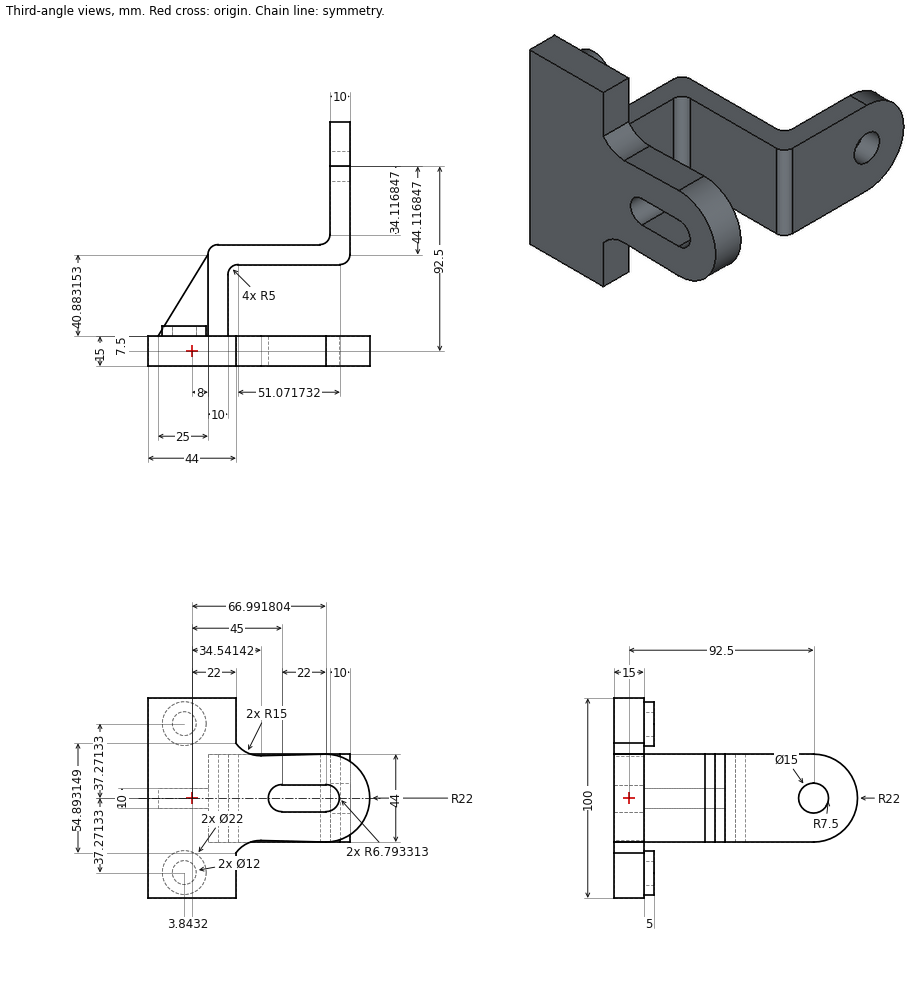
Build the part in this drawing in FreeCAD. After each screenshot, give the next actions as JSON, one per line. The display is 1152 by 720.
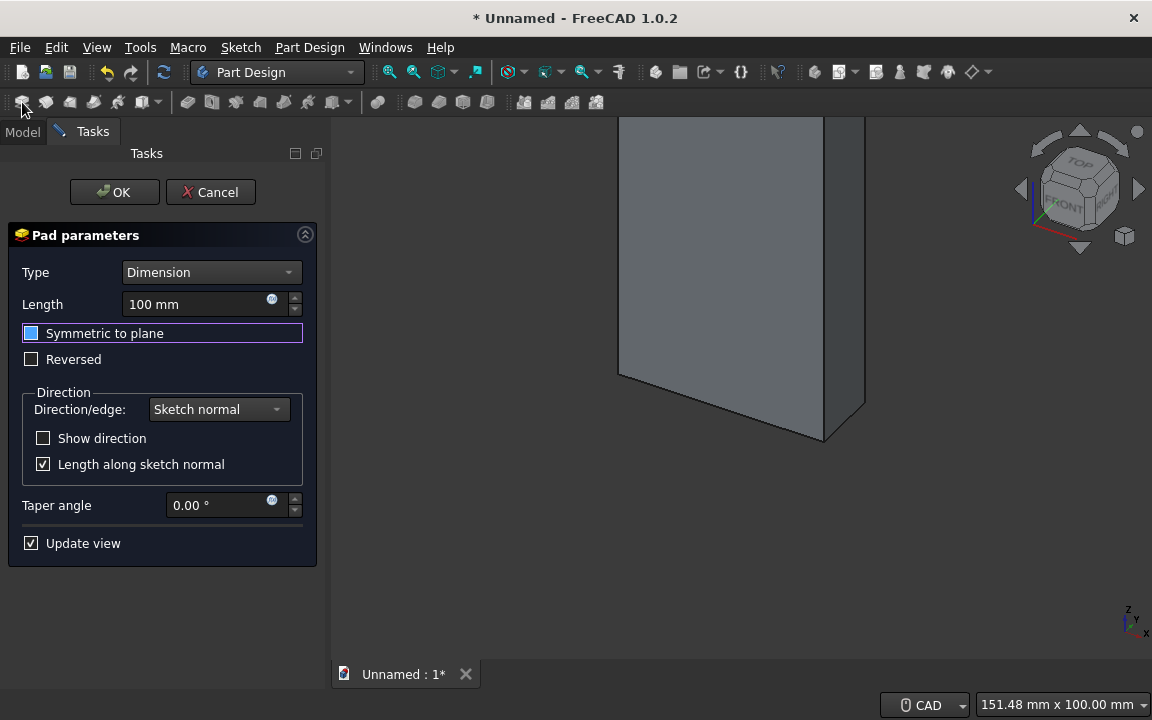
{"action": "left_click", "coordinate": [30, 333]}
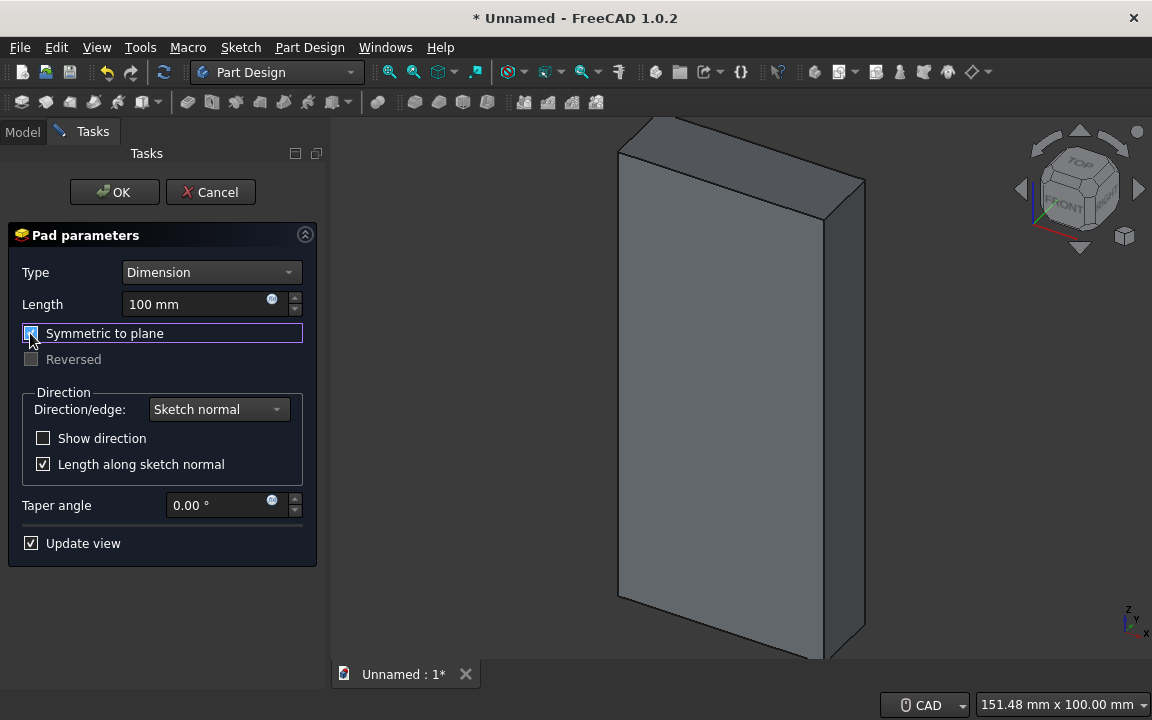
{"action": "left_click", "coordinate": [115, 192]}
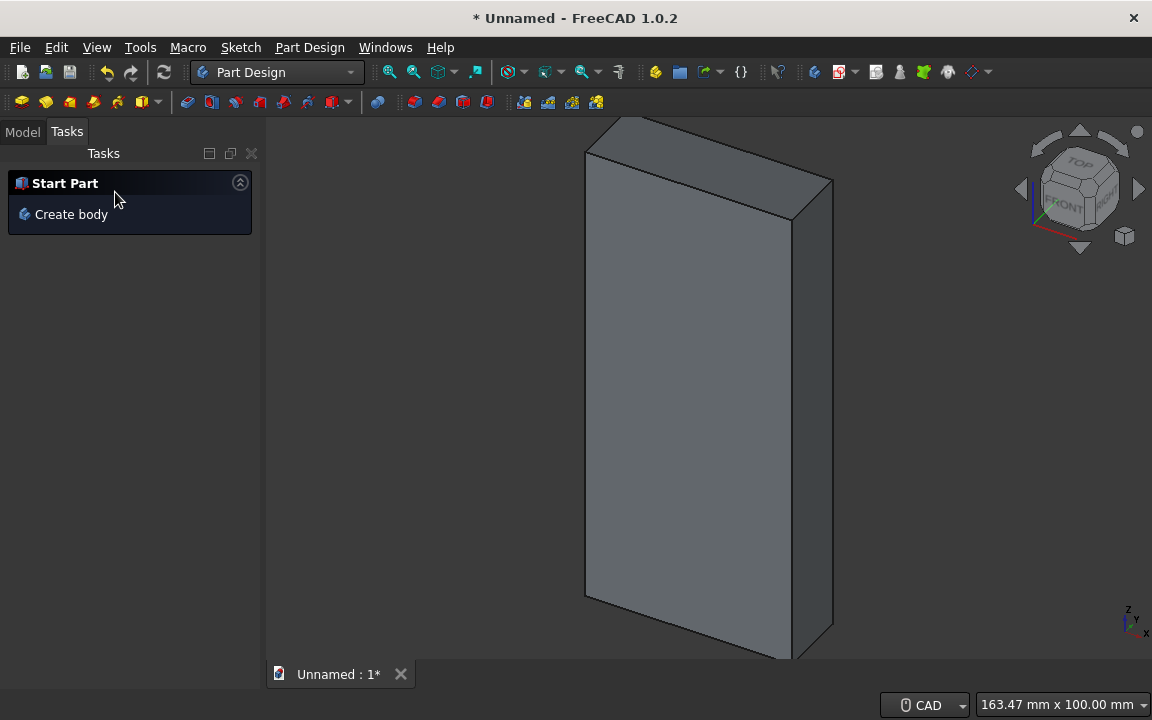
{"action": "left_click", "coordinate": [390, 72]}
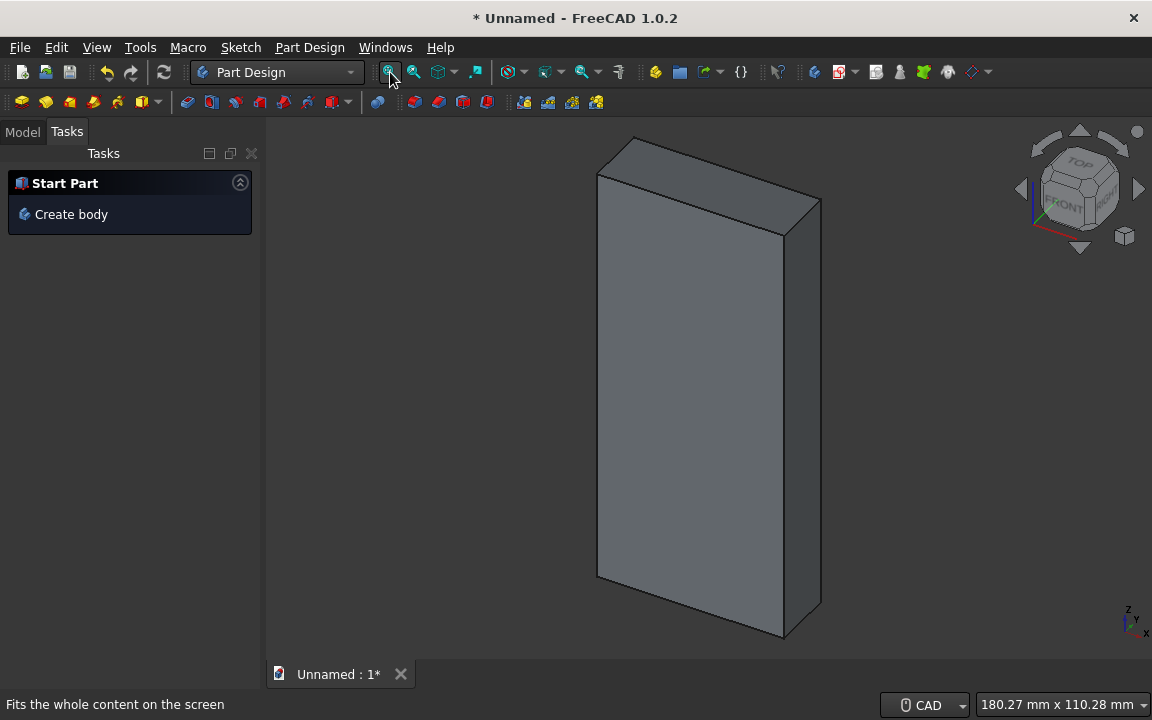
{"action": "left_click", "coordinate": [840, 72]}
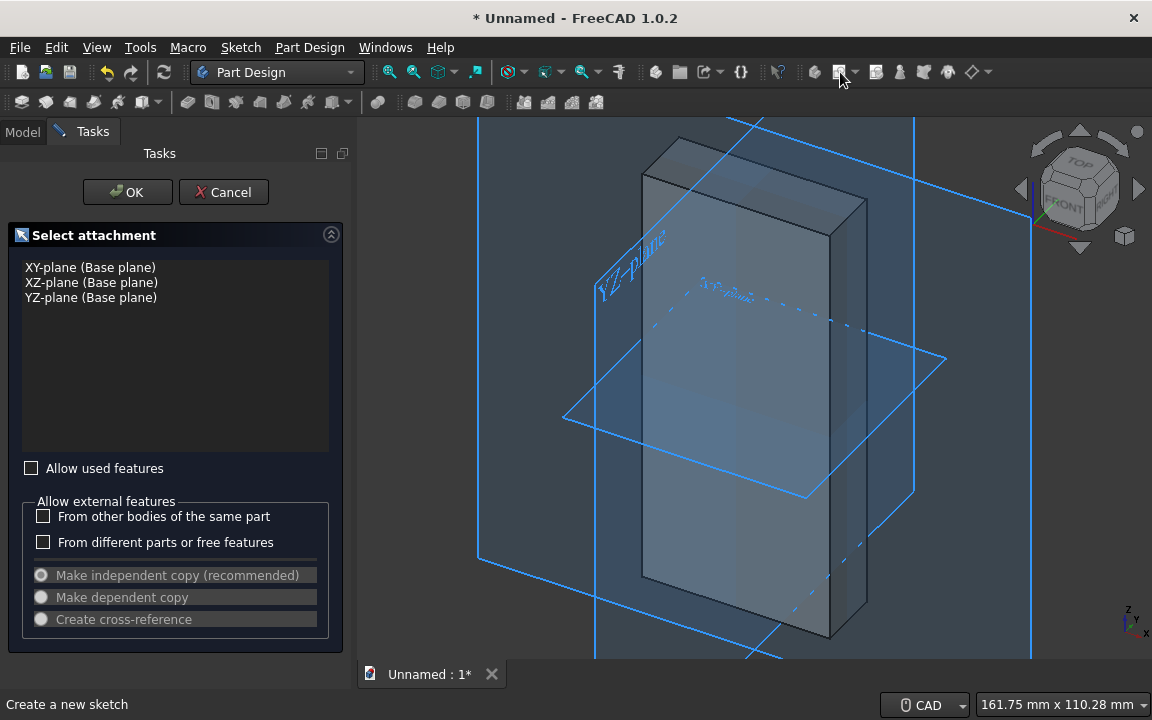
{"action": "left_click", "coordinate": [82, 268]}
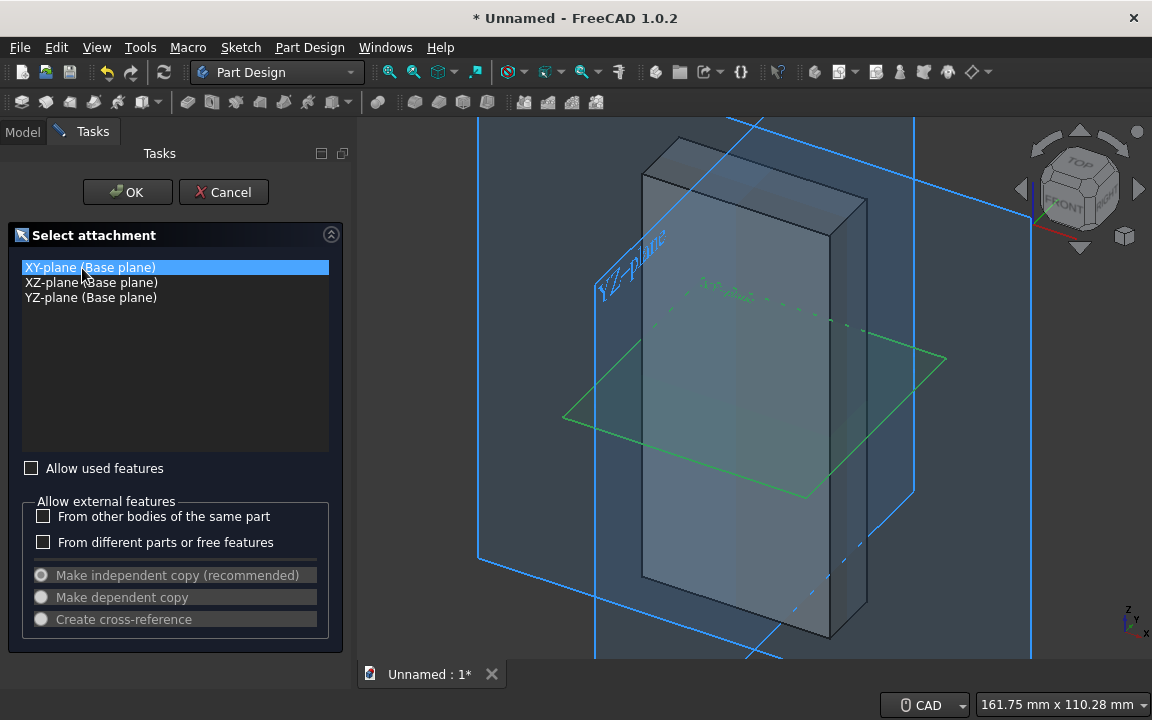
{"action": "left_click", "coordinate": [128, 192]}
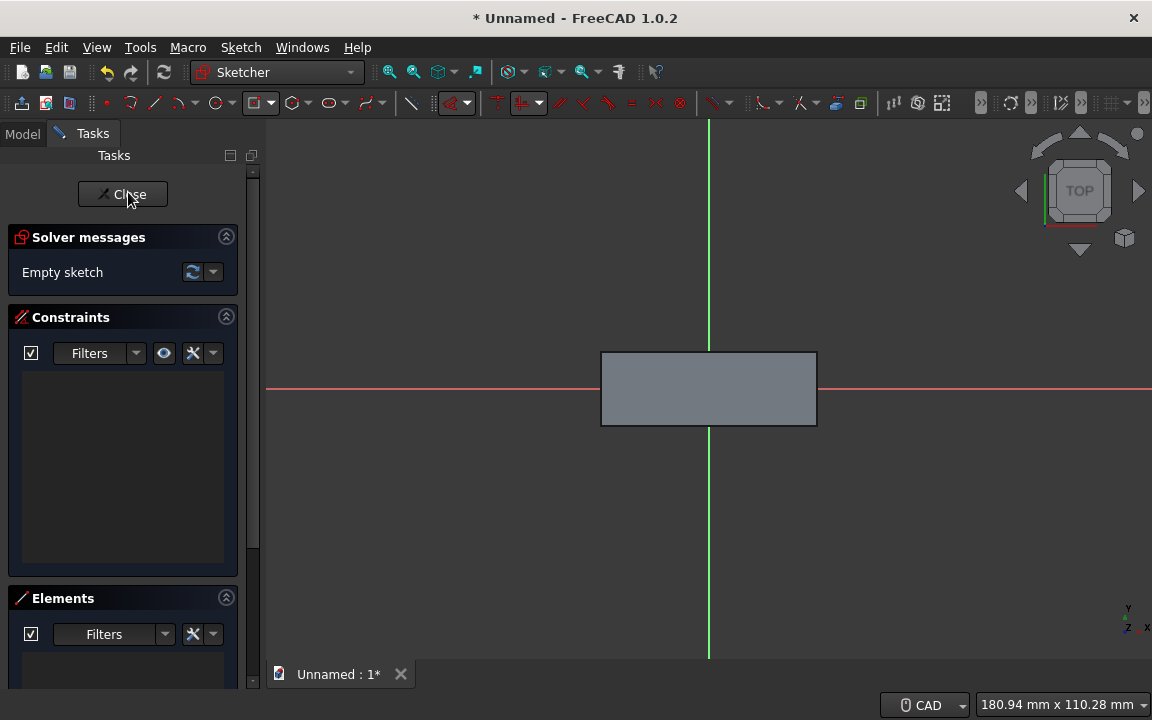
{"action": "left_click", "coordinate": [70, 104]}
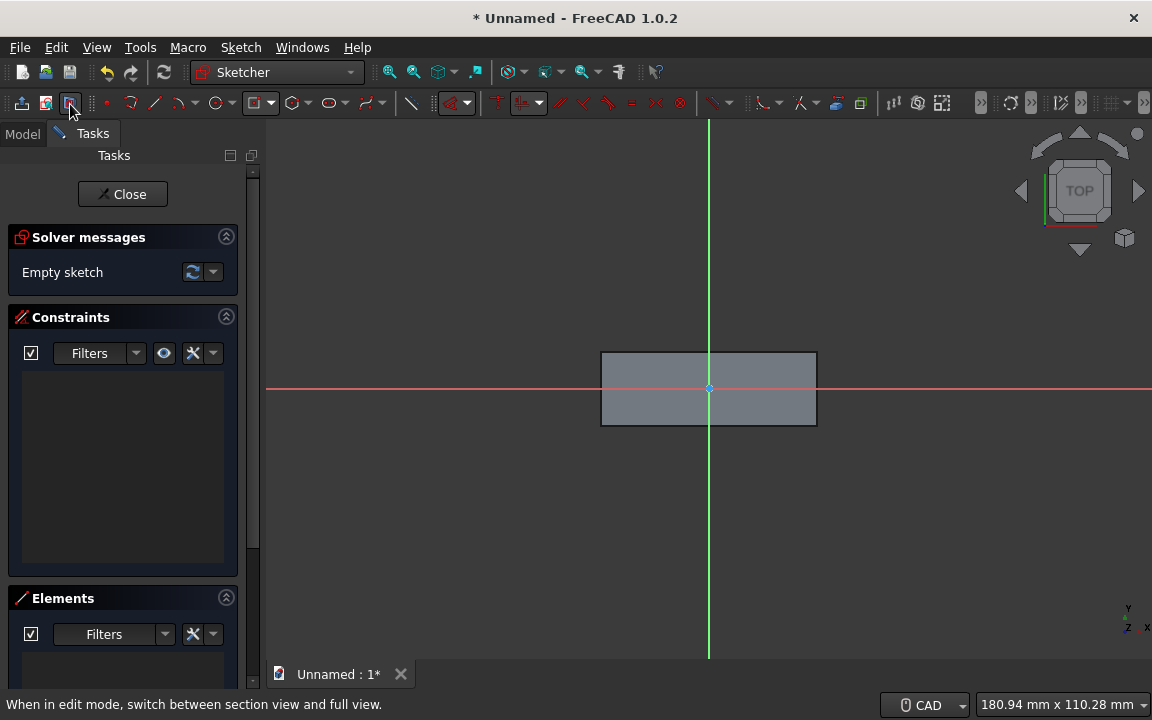
{"action": "scroll", "coordinate": [322, 631], "scroll_direction": "down", "scroll_amount": 3}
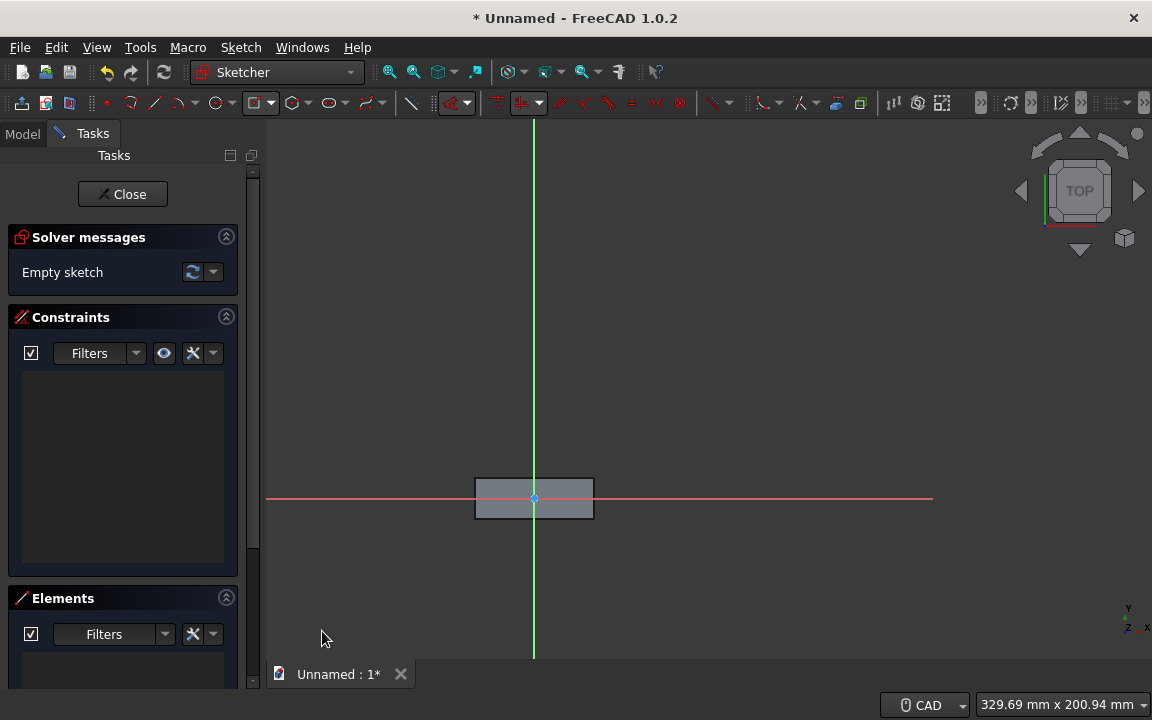
{"action": "scroll", "coordinate": [641, 344], "scroll_direction": "up", "scroll_amount": 2}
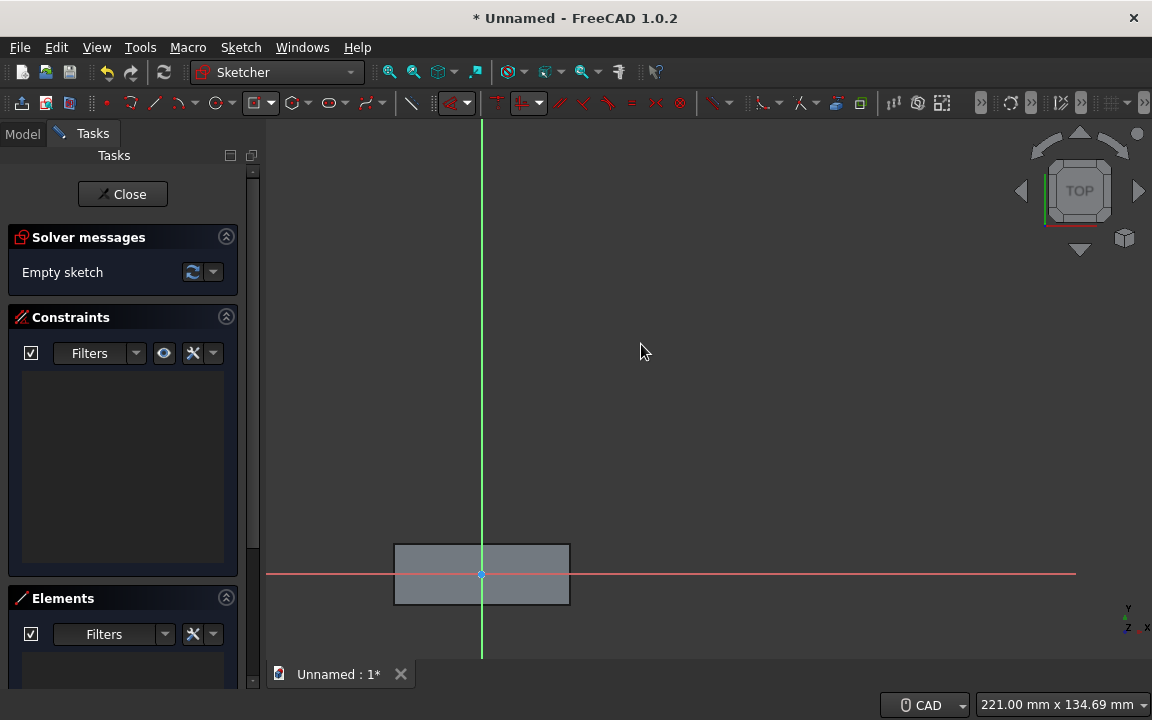
{"action": "left_click", "coordinate": [156, 104]}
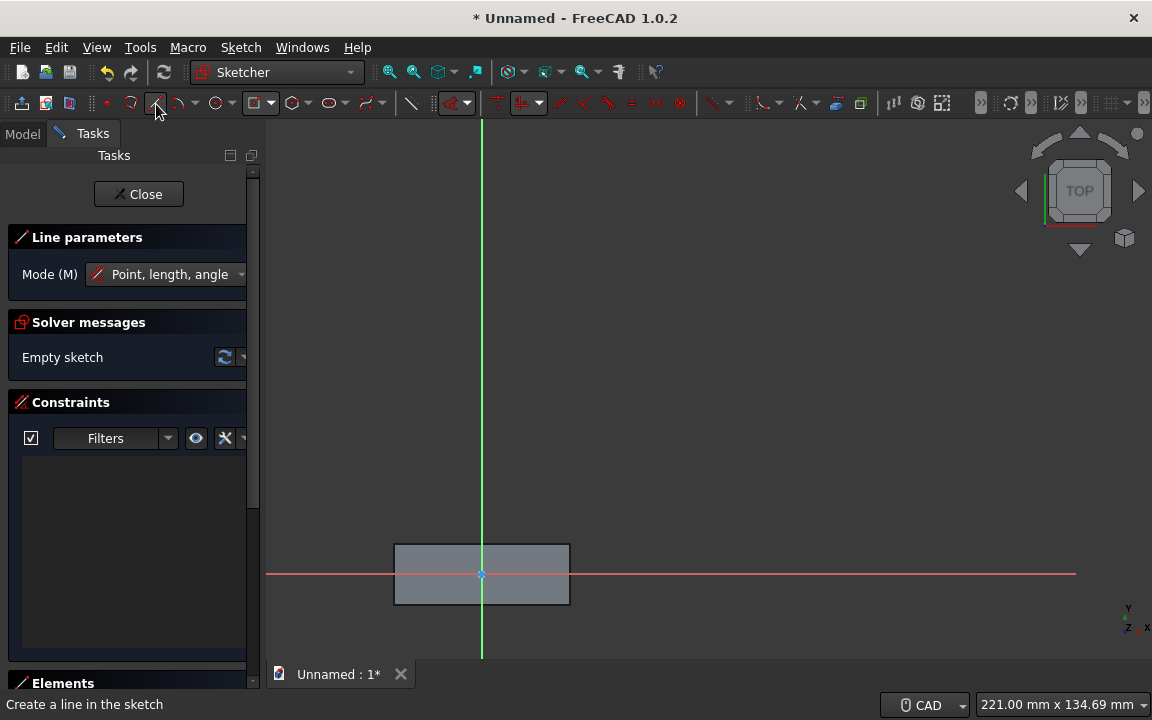
{"action": "left_click", "coordinate": [574, 401]}
{"action": "left_click", "coordinate": [779, 401]}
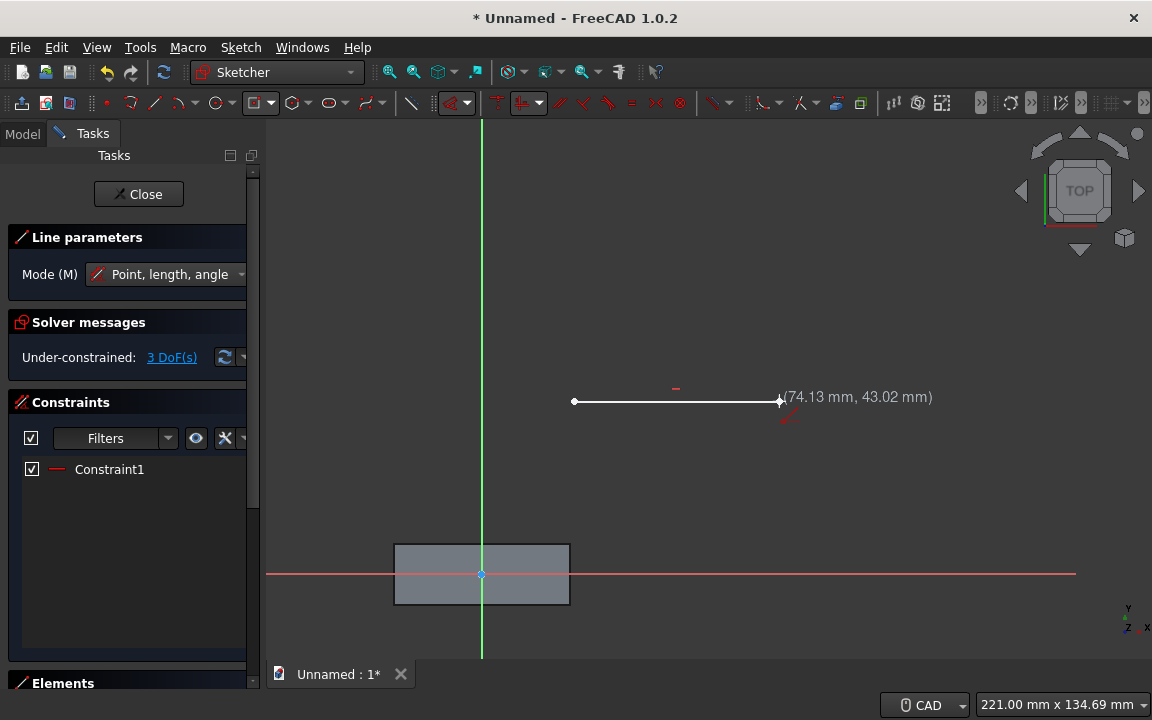
{"action": "left_click", "coordinate": [132, 104]}